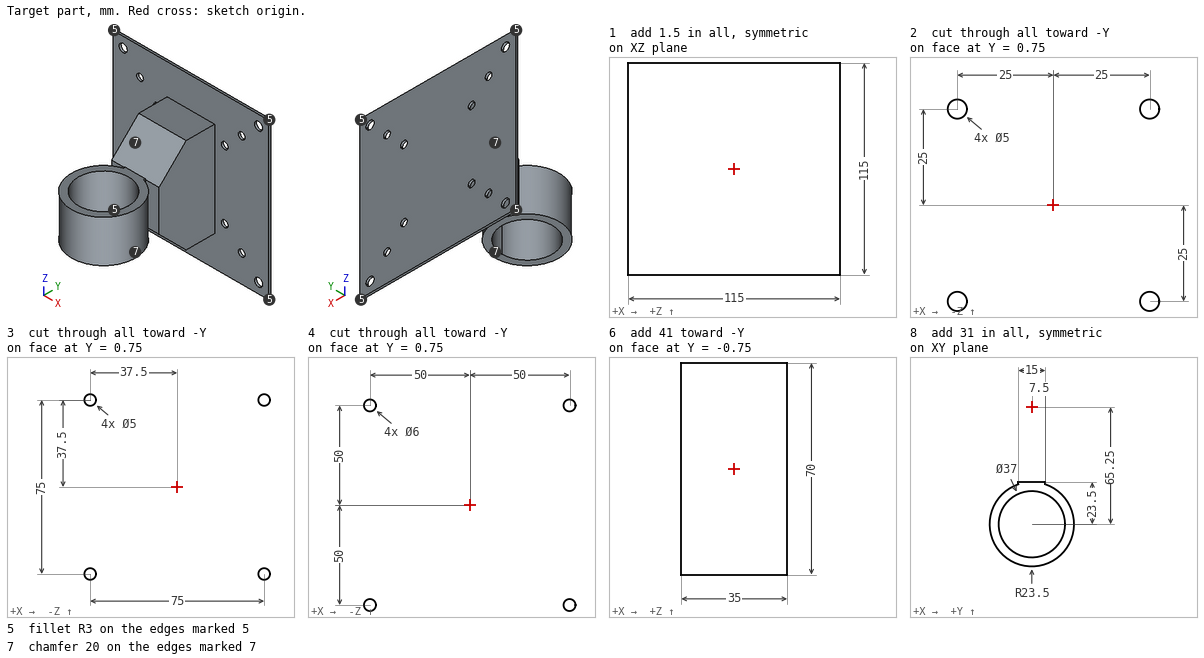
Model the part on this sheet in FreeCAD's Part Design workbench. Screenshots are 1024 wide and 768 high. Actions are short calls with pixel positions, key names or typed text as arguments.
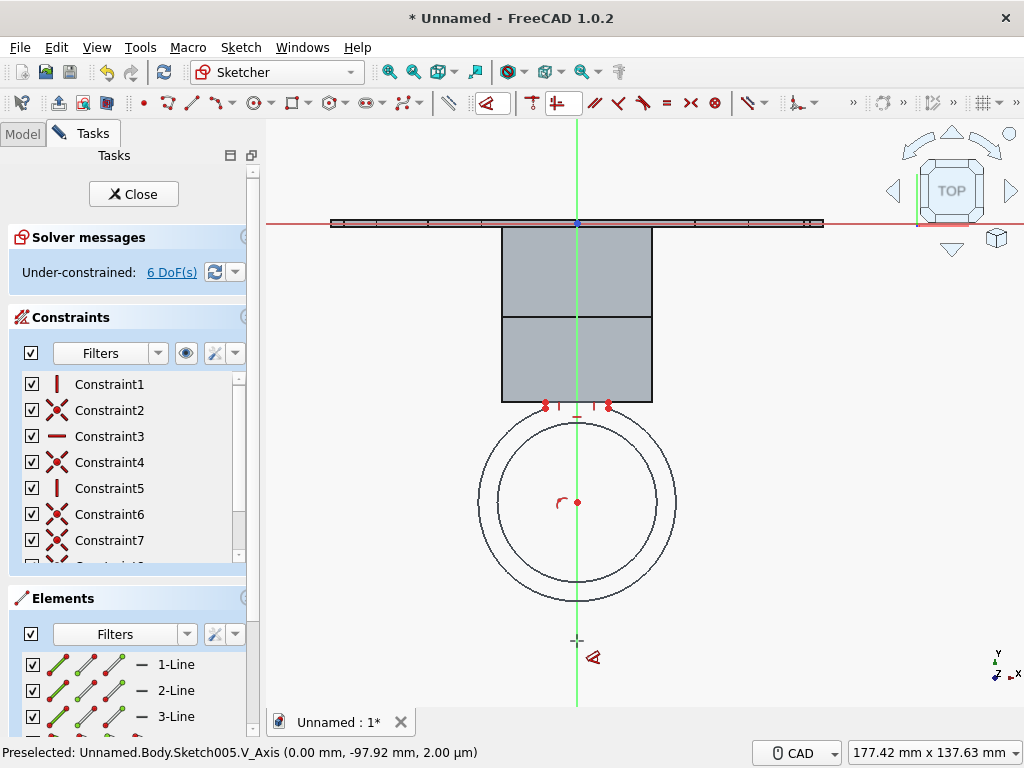
click(488, 545)
click(459, 559)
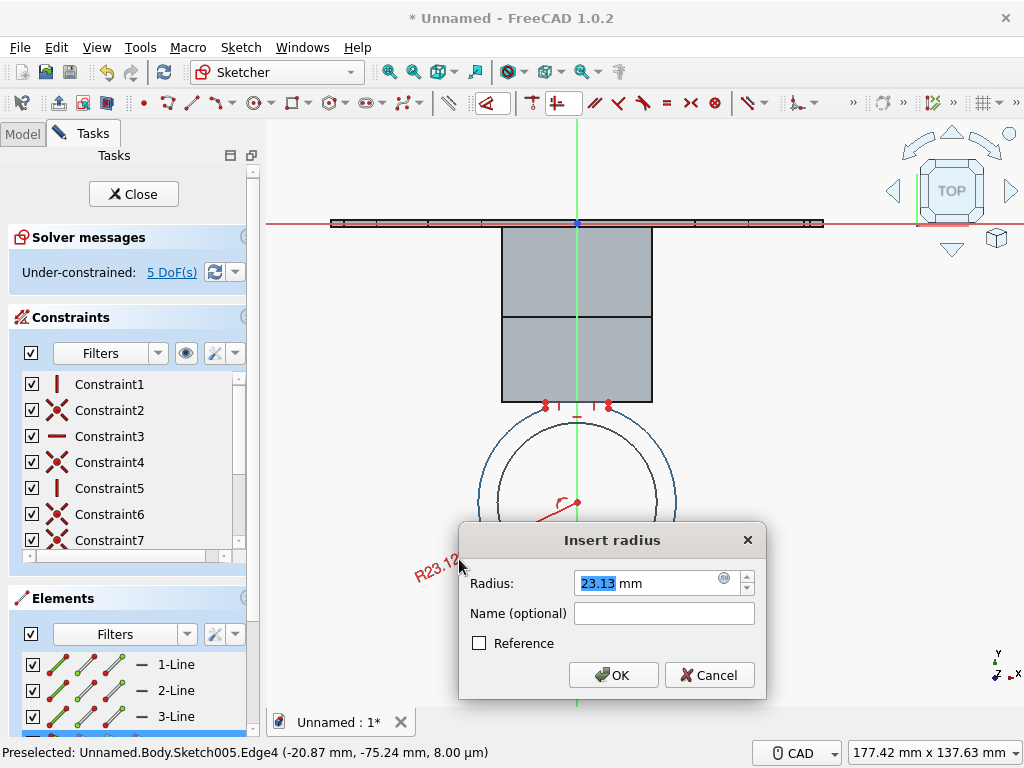
text(23.5)
key(Return)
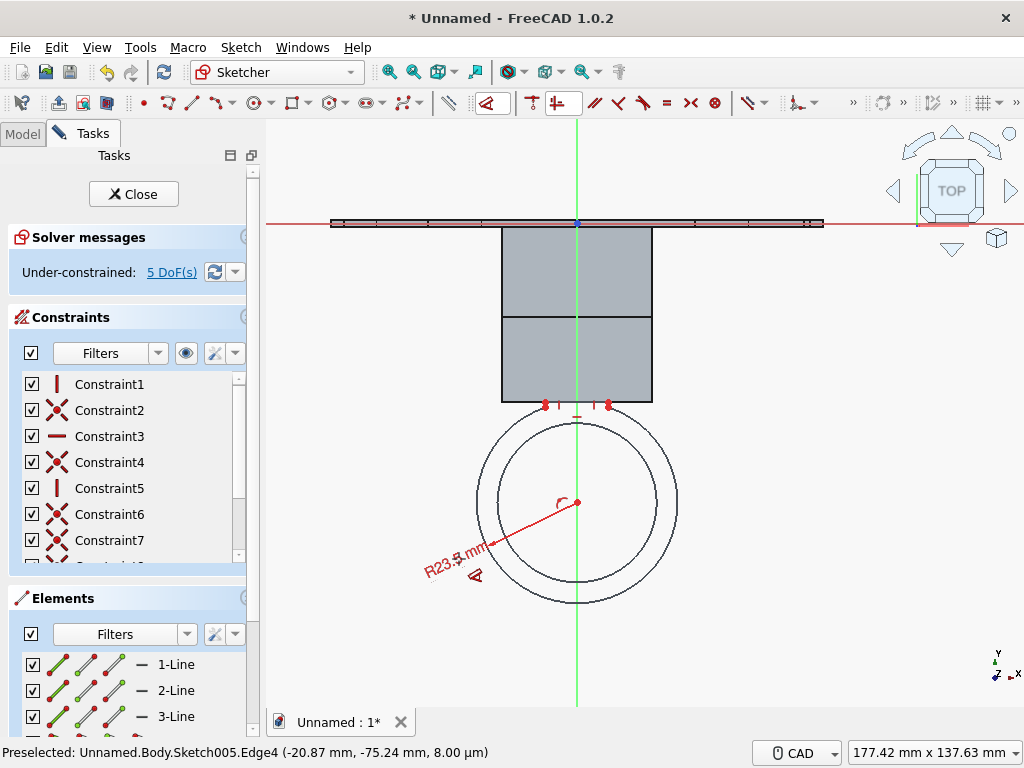
click(633, 446)
click(672, 407)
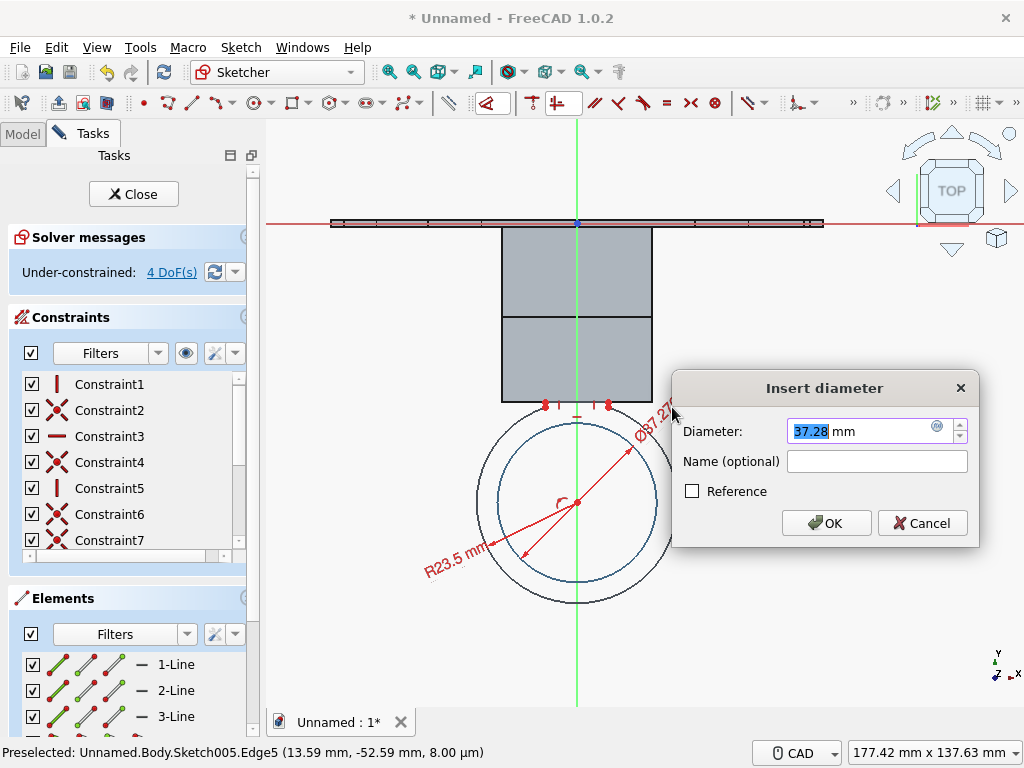
text(37)
key(Return)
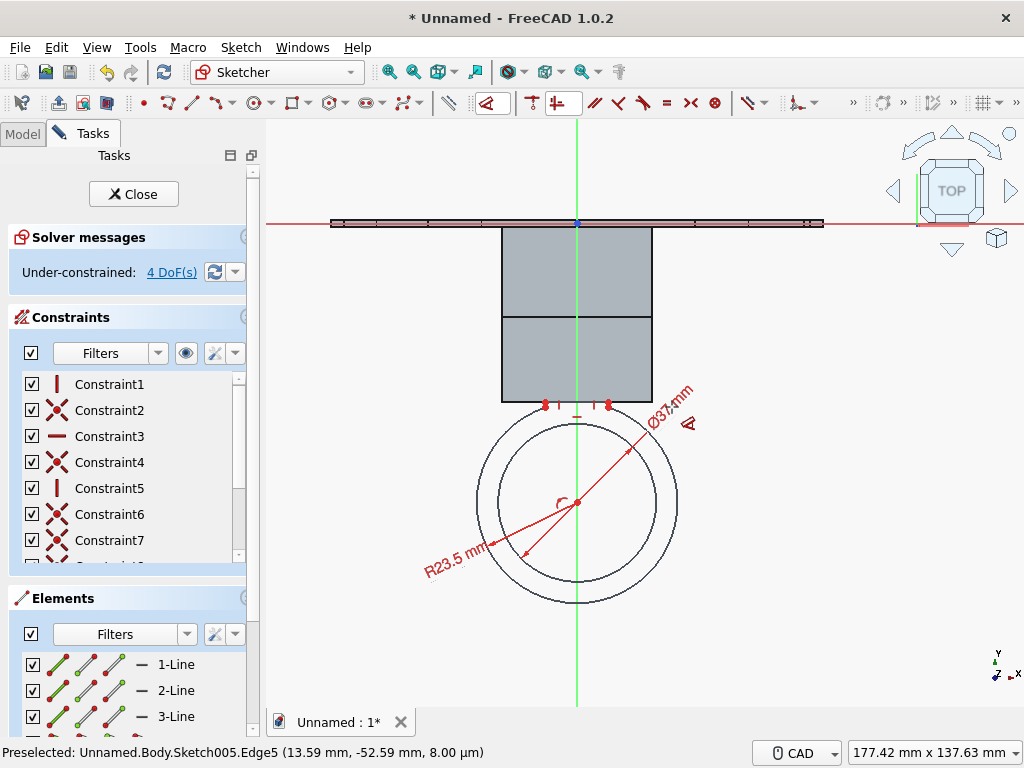
click(590, 402)
click(562, 368)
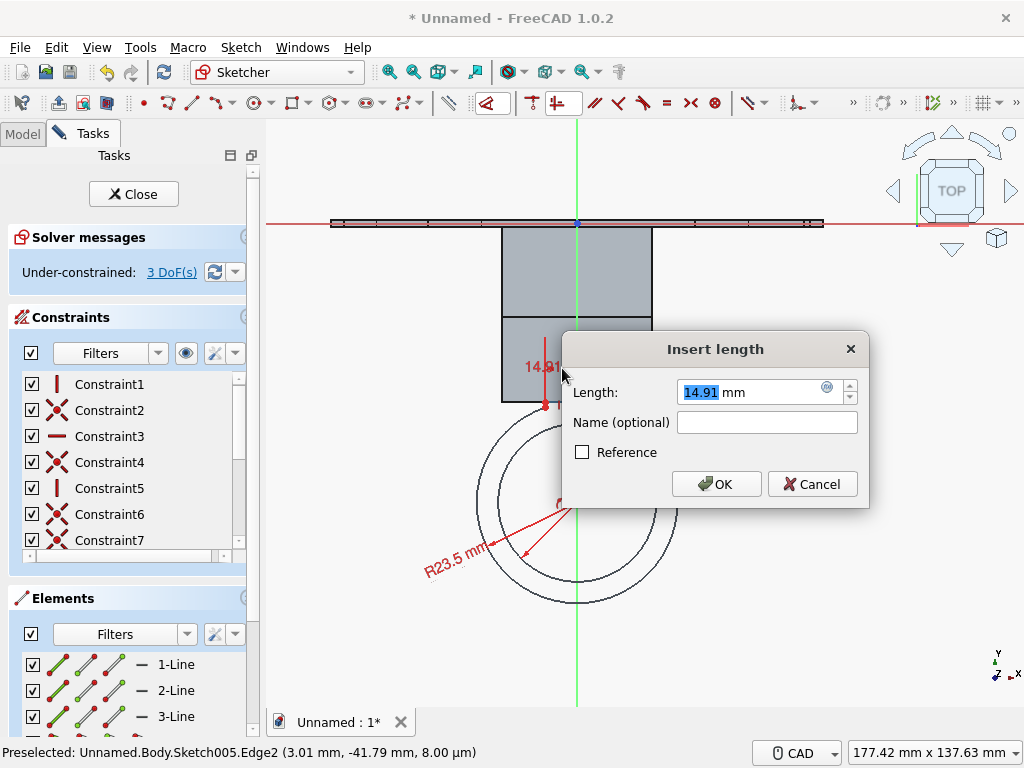
text(15)
key(Return)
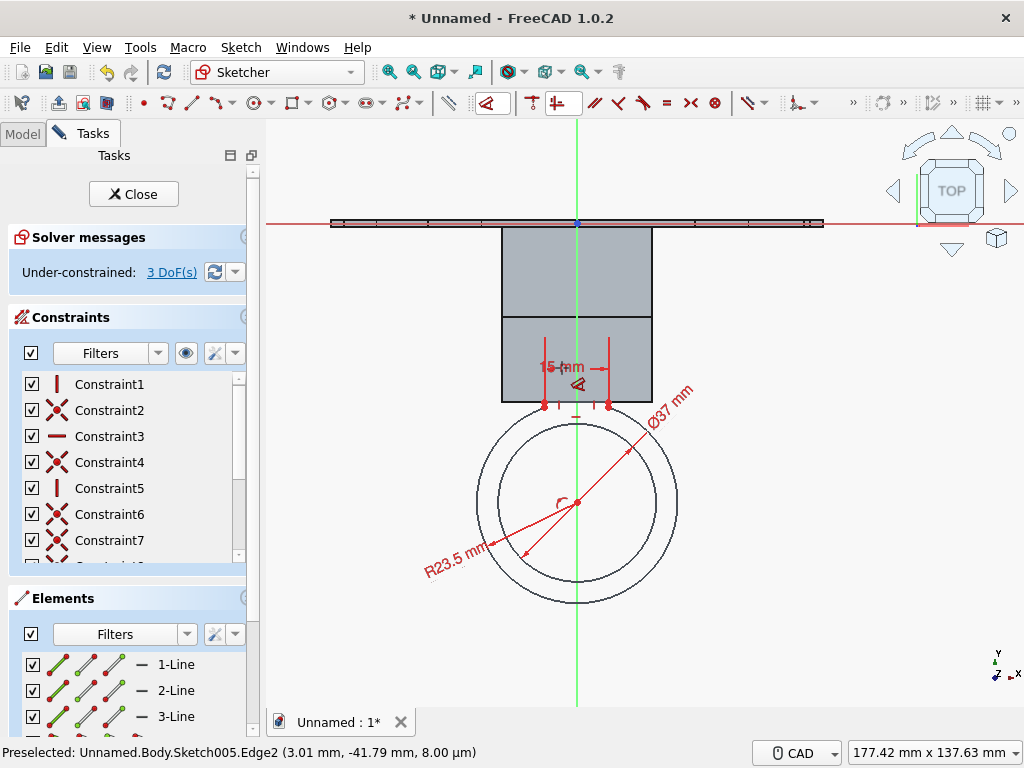
scroll(609, 408, up, 5)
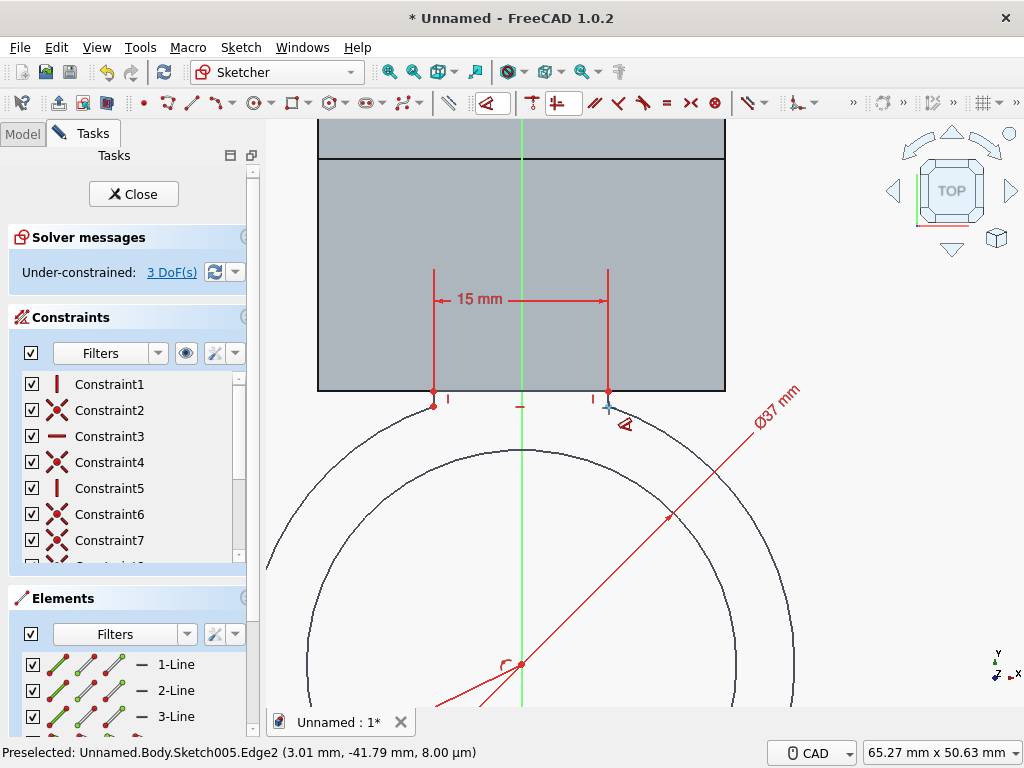
click(608, 406)
click(565, 440)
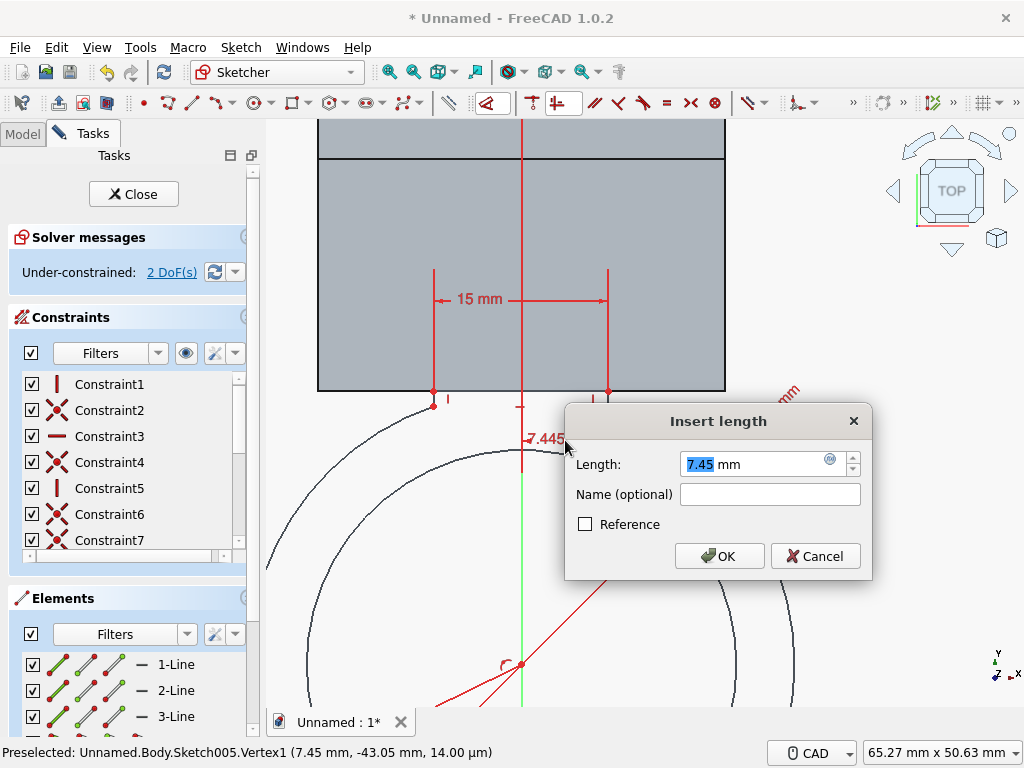
text(7.5)
key(Return)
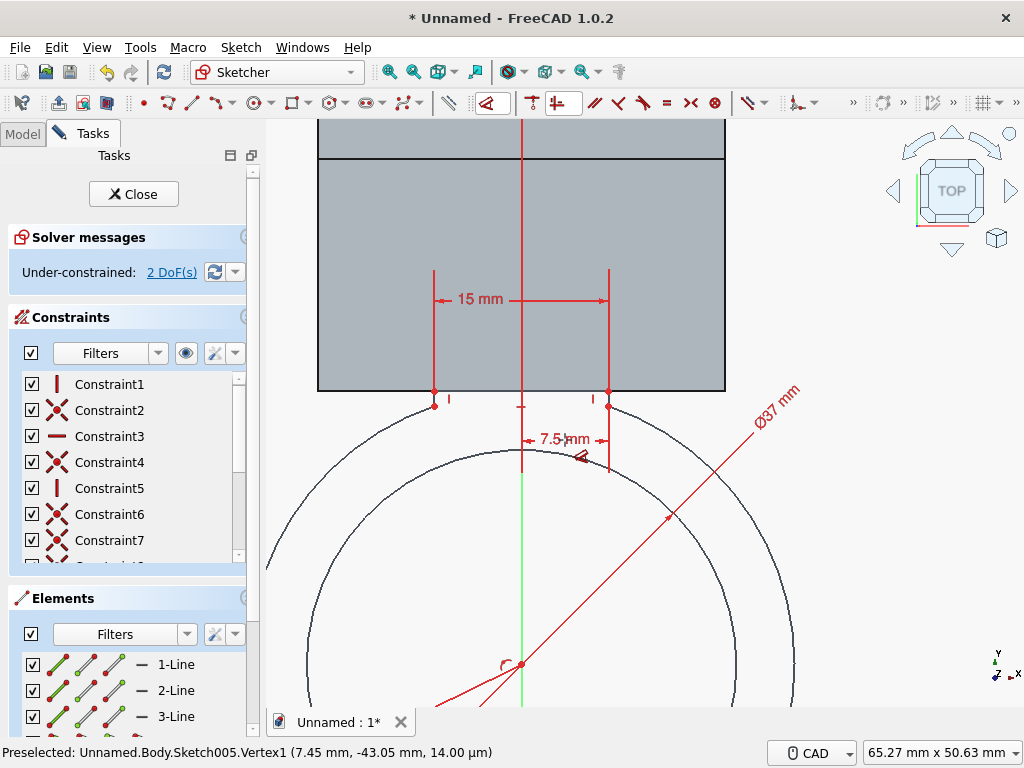
click(522, 665)
click(556, 406)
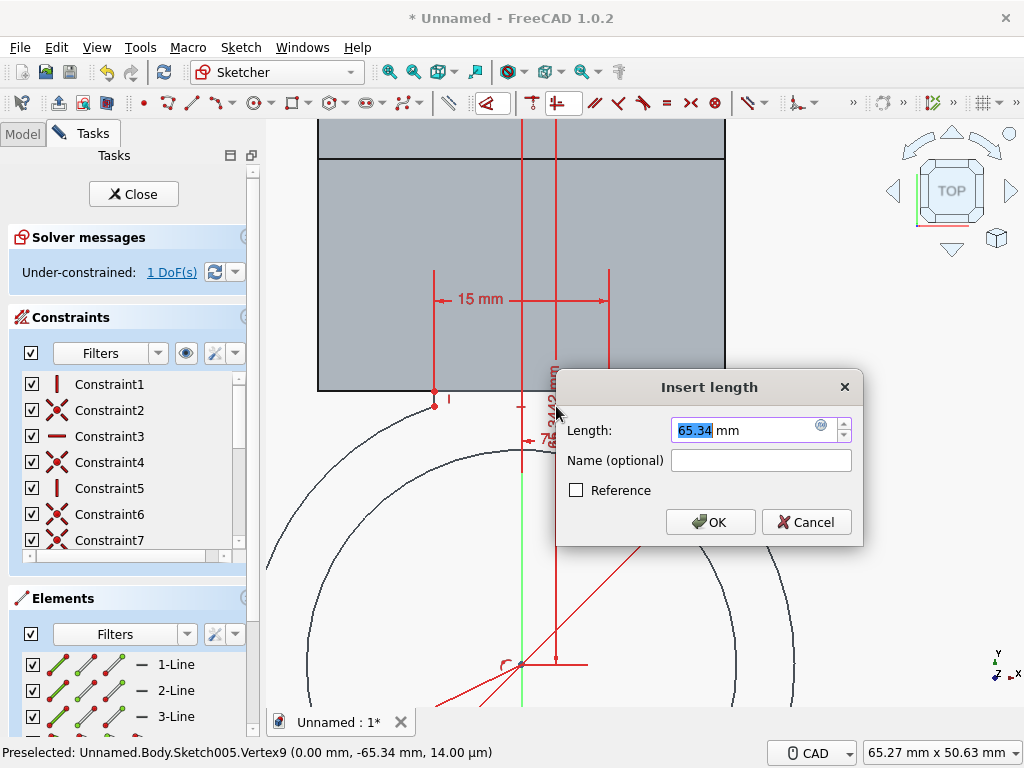
text(65.25)
key(Return)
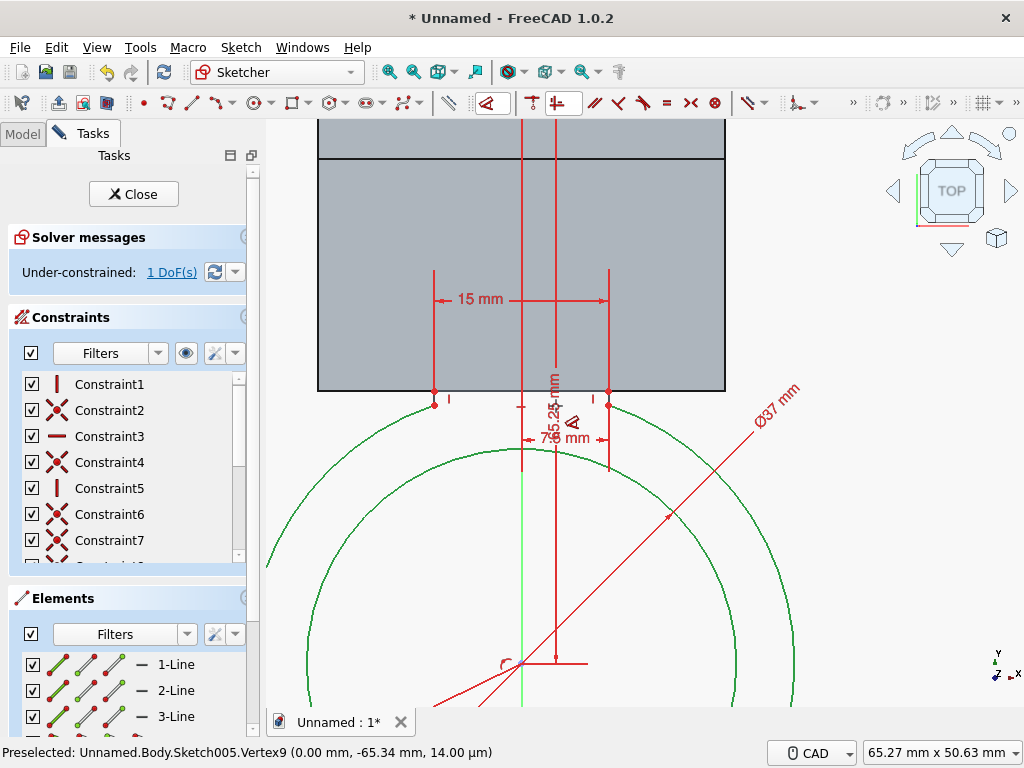
click(609, 391)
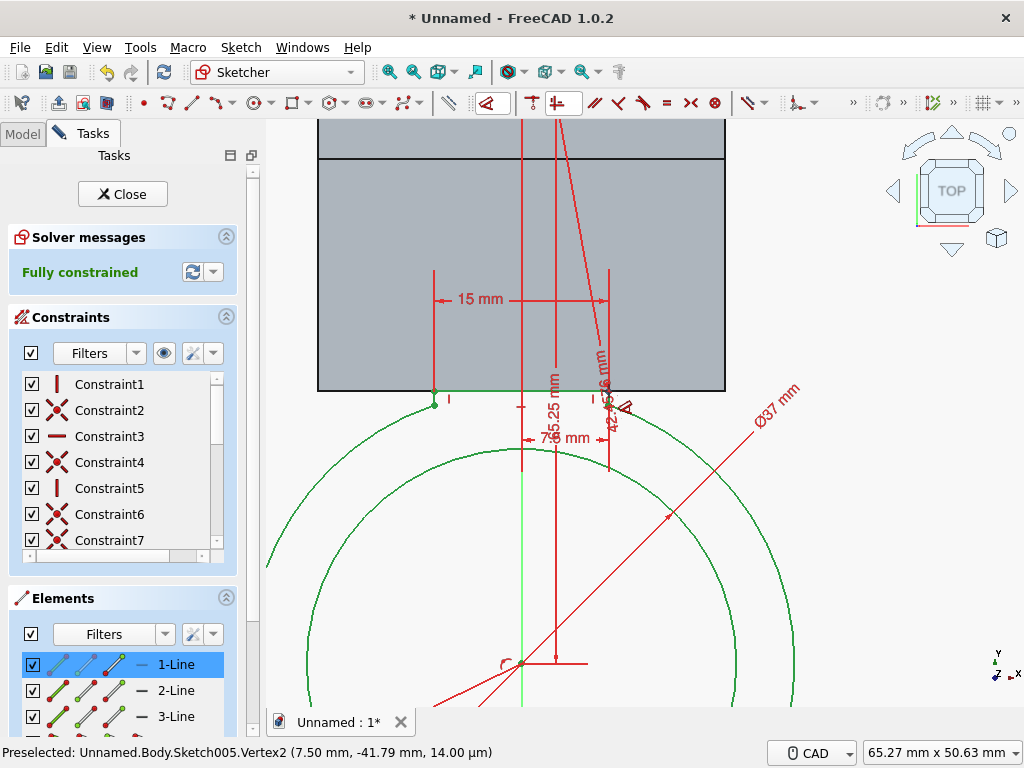
click(522, 664)
click(643, 528)